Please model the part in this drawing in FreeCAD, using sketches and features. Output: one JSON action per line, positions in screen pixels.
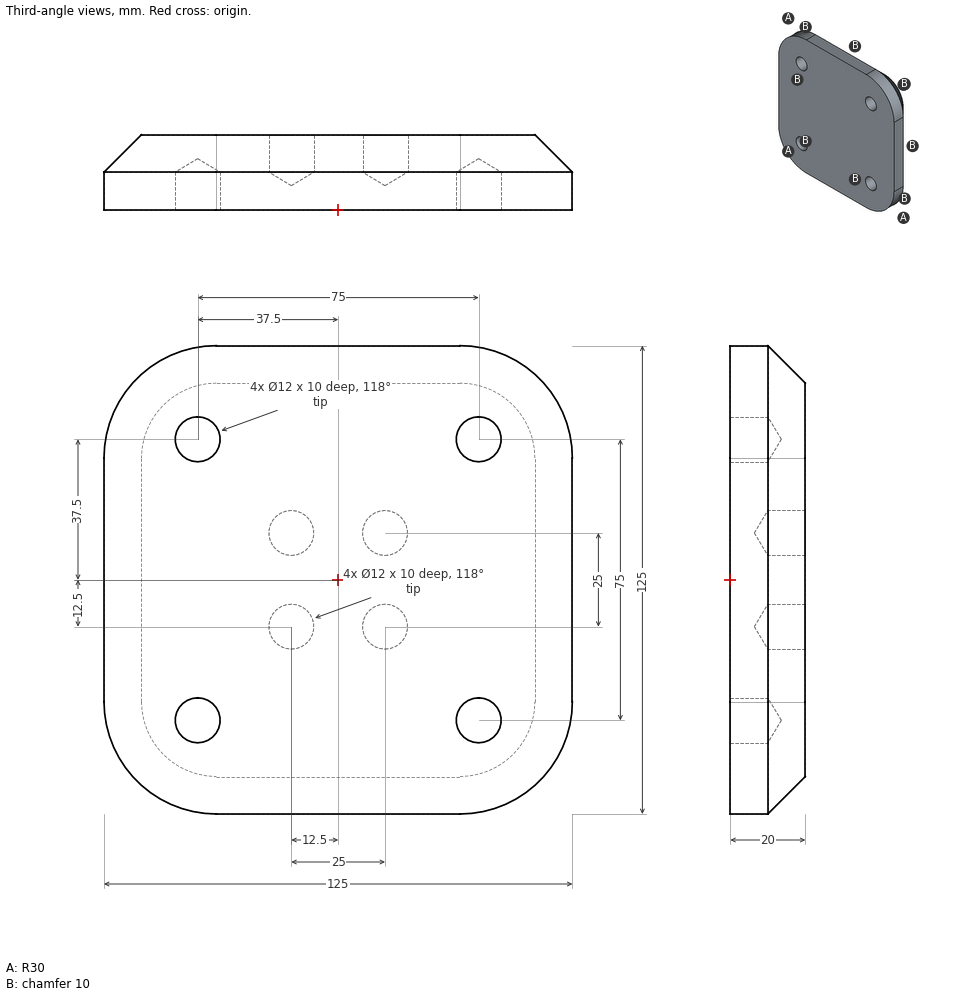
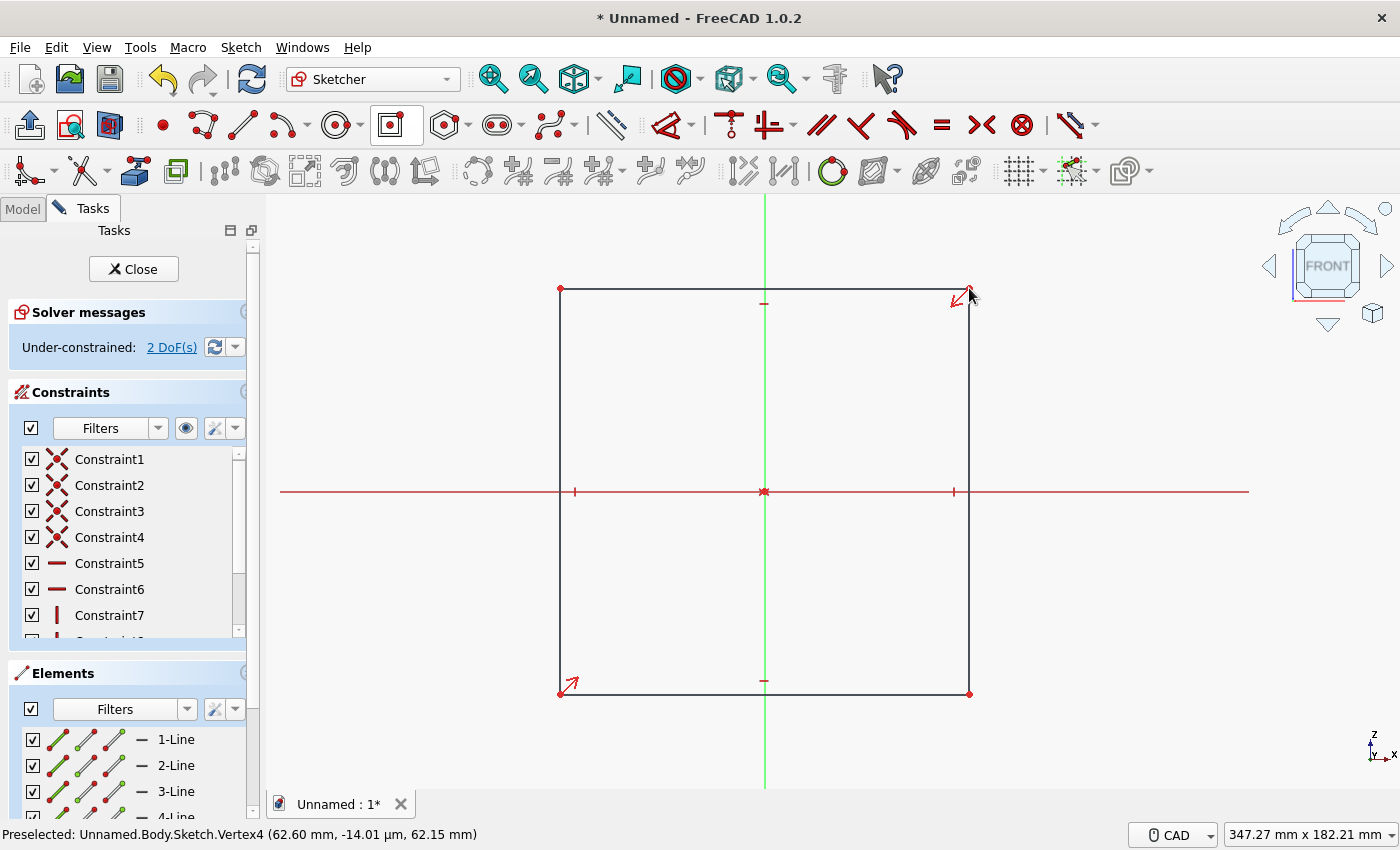
{"action": "key", "text": "d"}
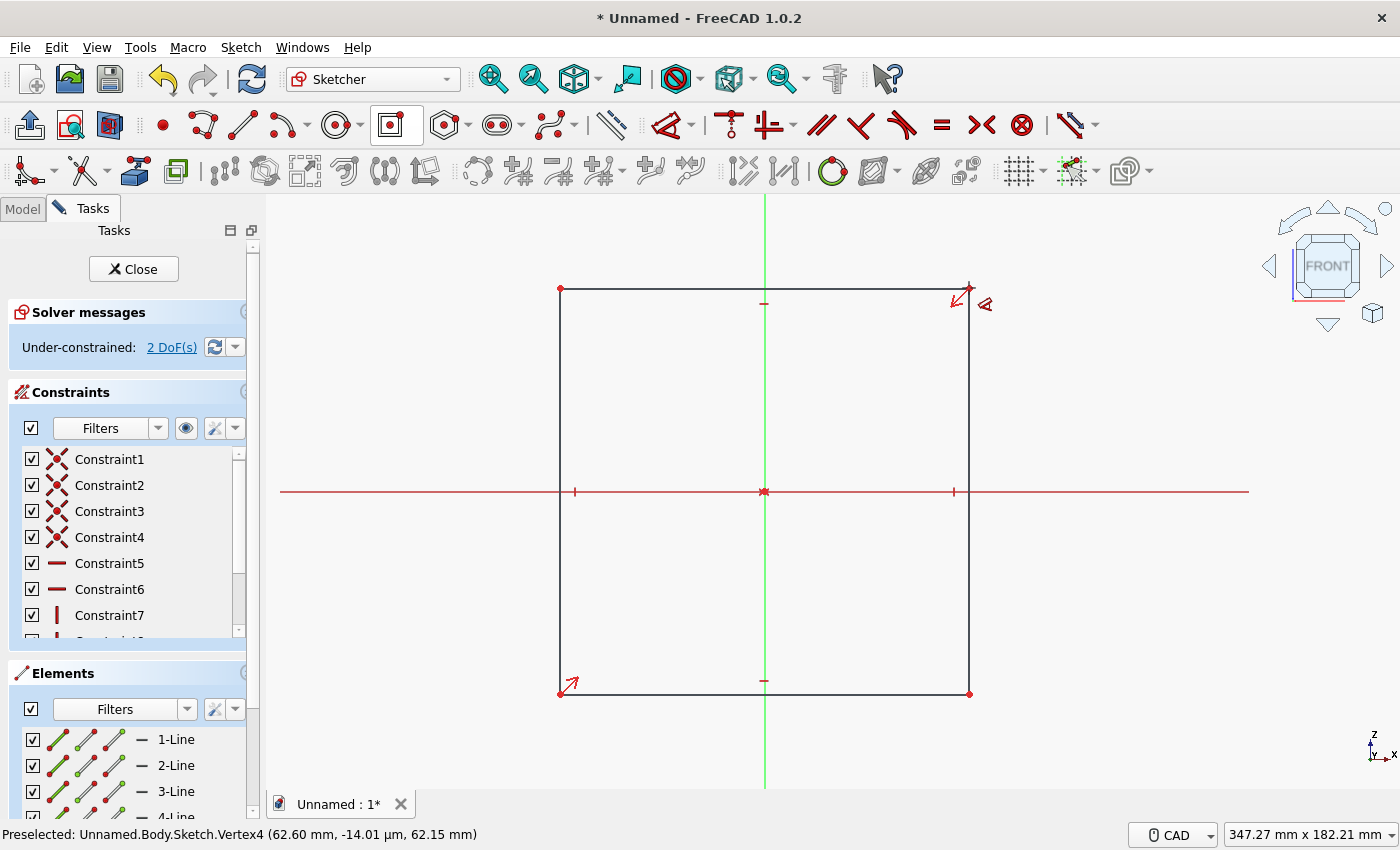
{"action": "left_click", "coordinate": [683, 695]}
{"action": "left_click", "coordinate": [671, 729]}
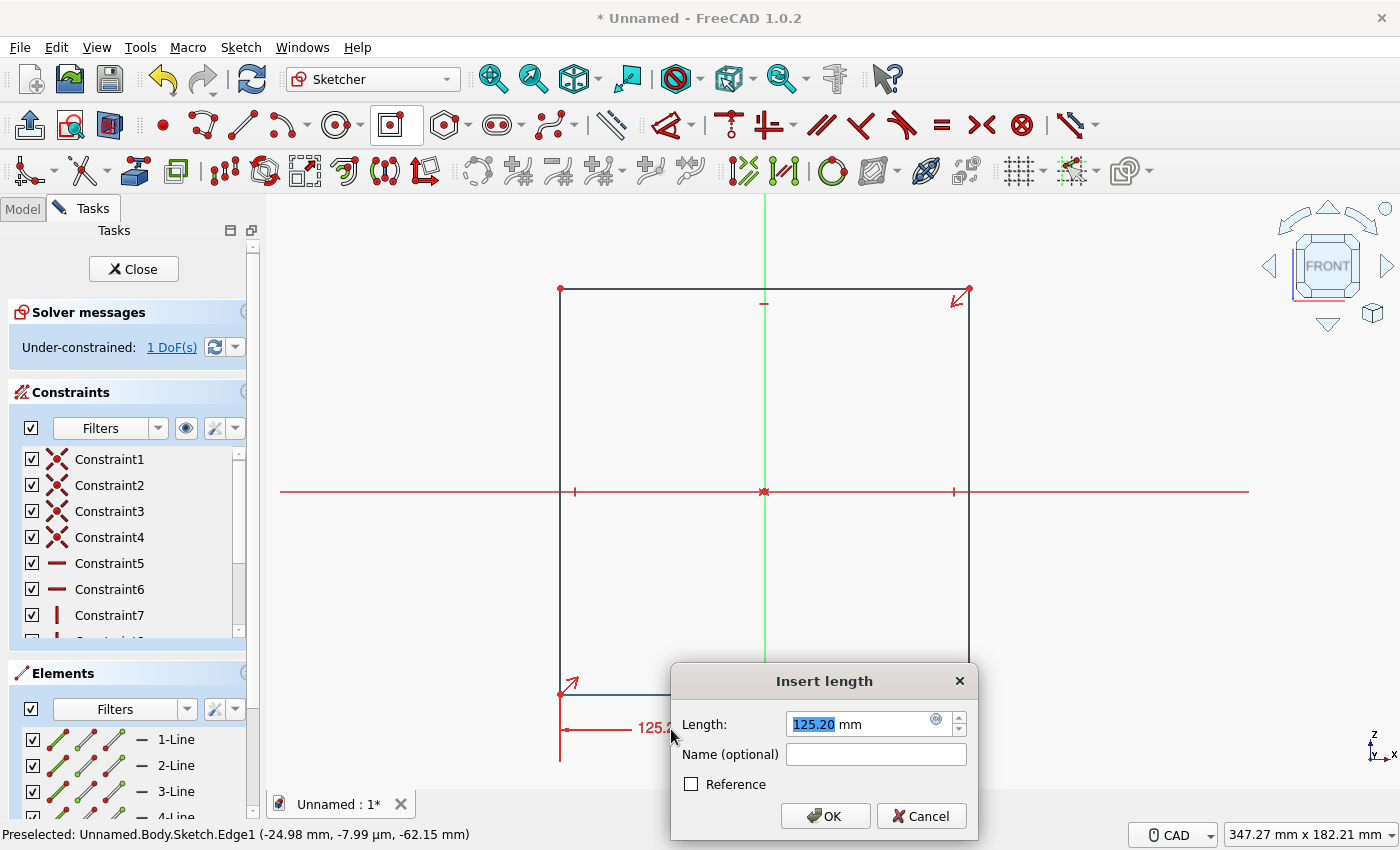
{"action": "type", "text": "125"}
{"action": "key", "text": "Return"}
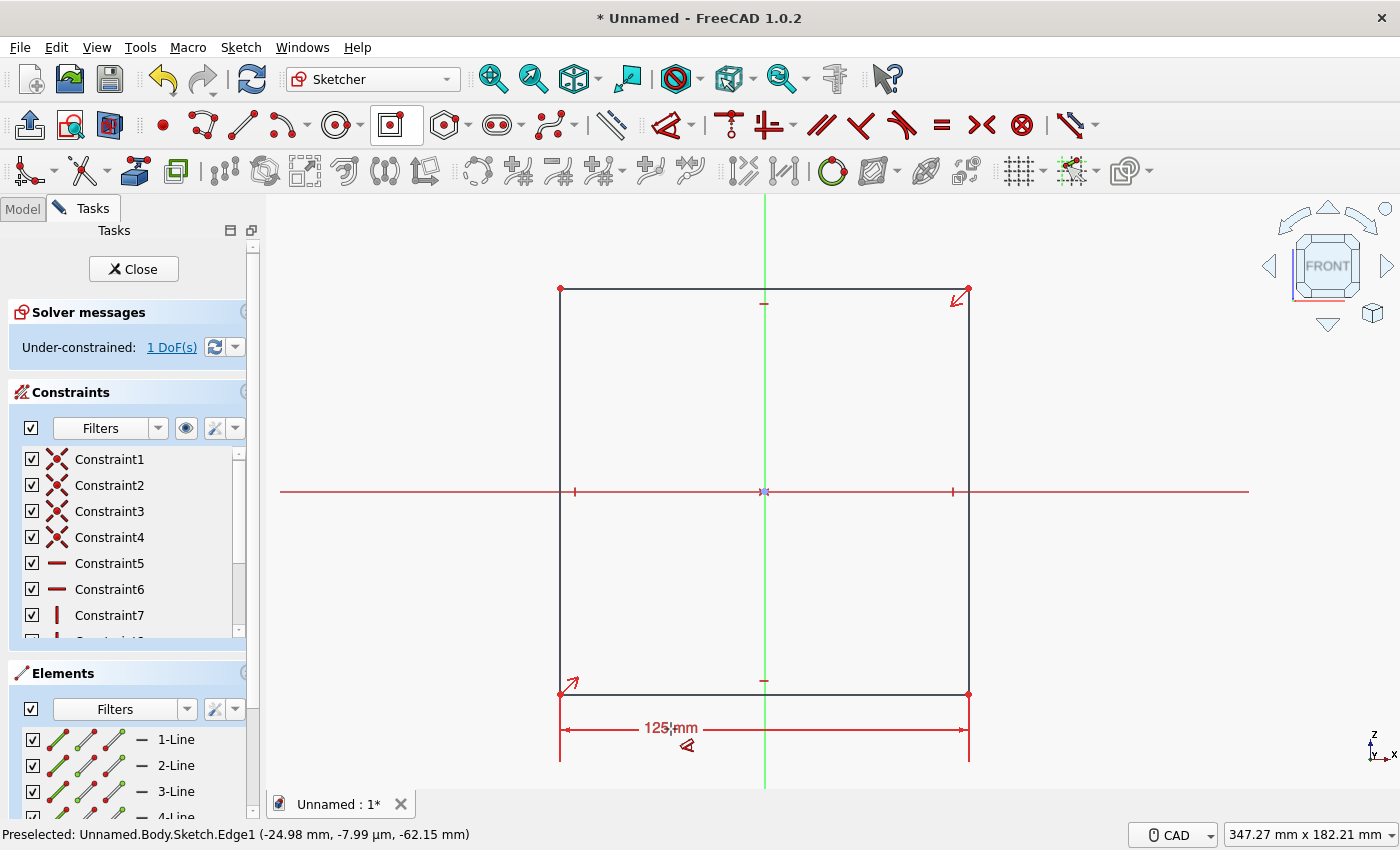
{"action": "left_click", "coordinate": [969, 573]}
{"action": "left_click", "coordinate": [1003, 399]}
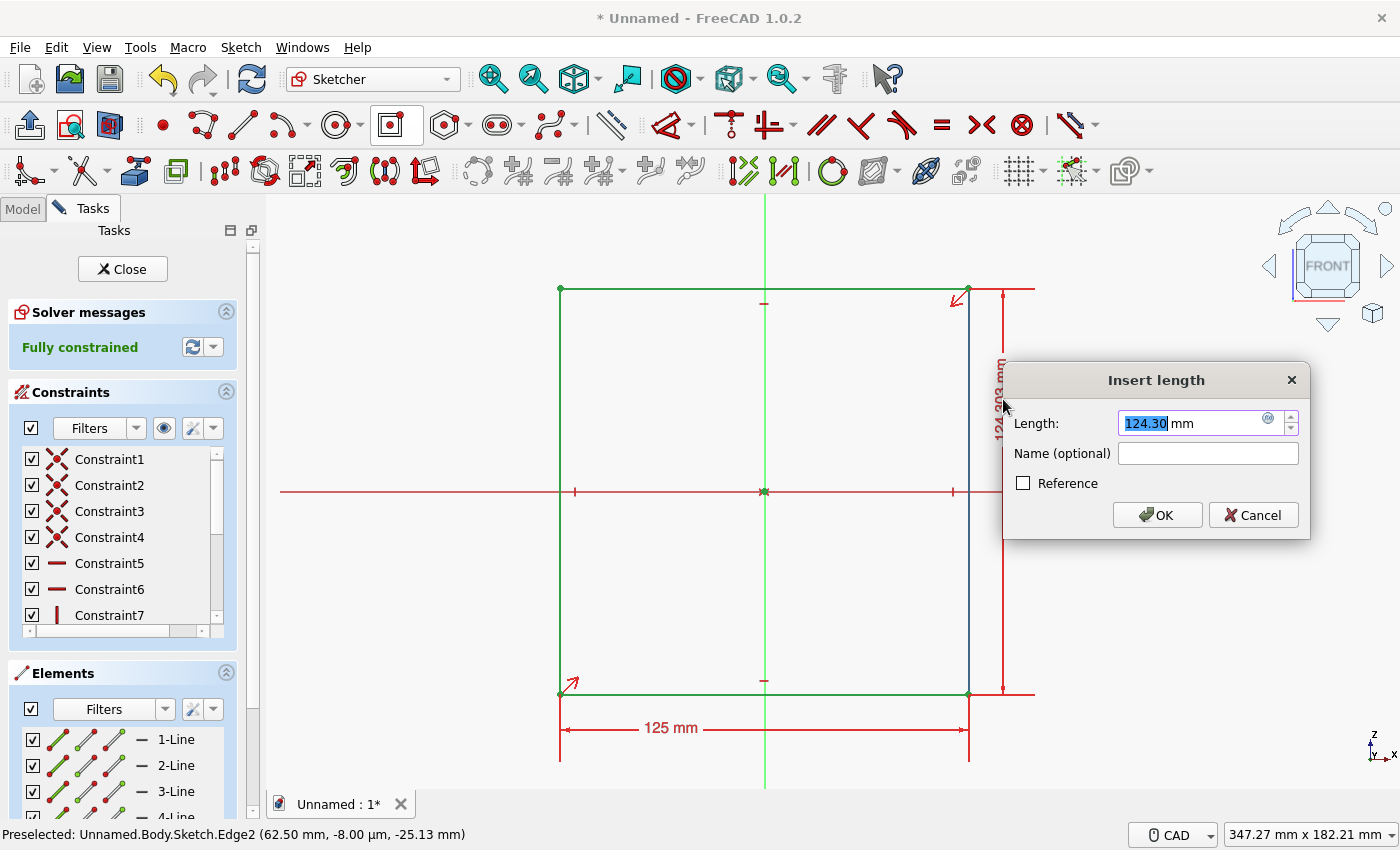
{"action": "type", "text": "125"}
{"action": "key", "text": "Return"}
{"action": "key", "text": "Escape"}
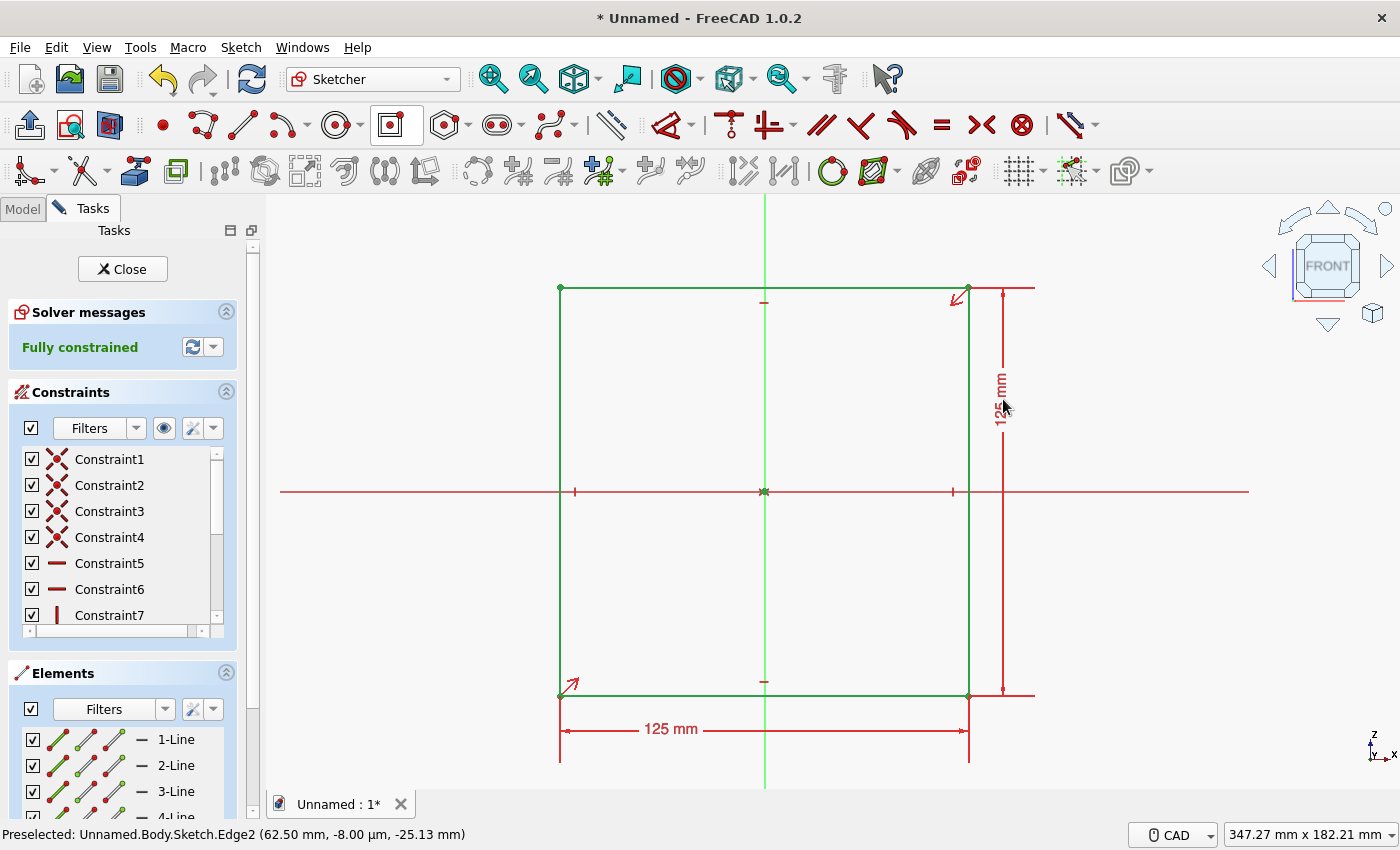
{"action": "left_click", "coordinate": [123, 269]}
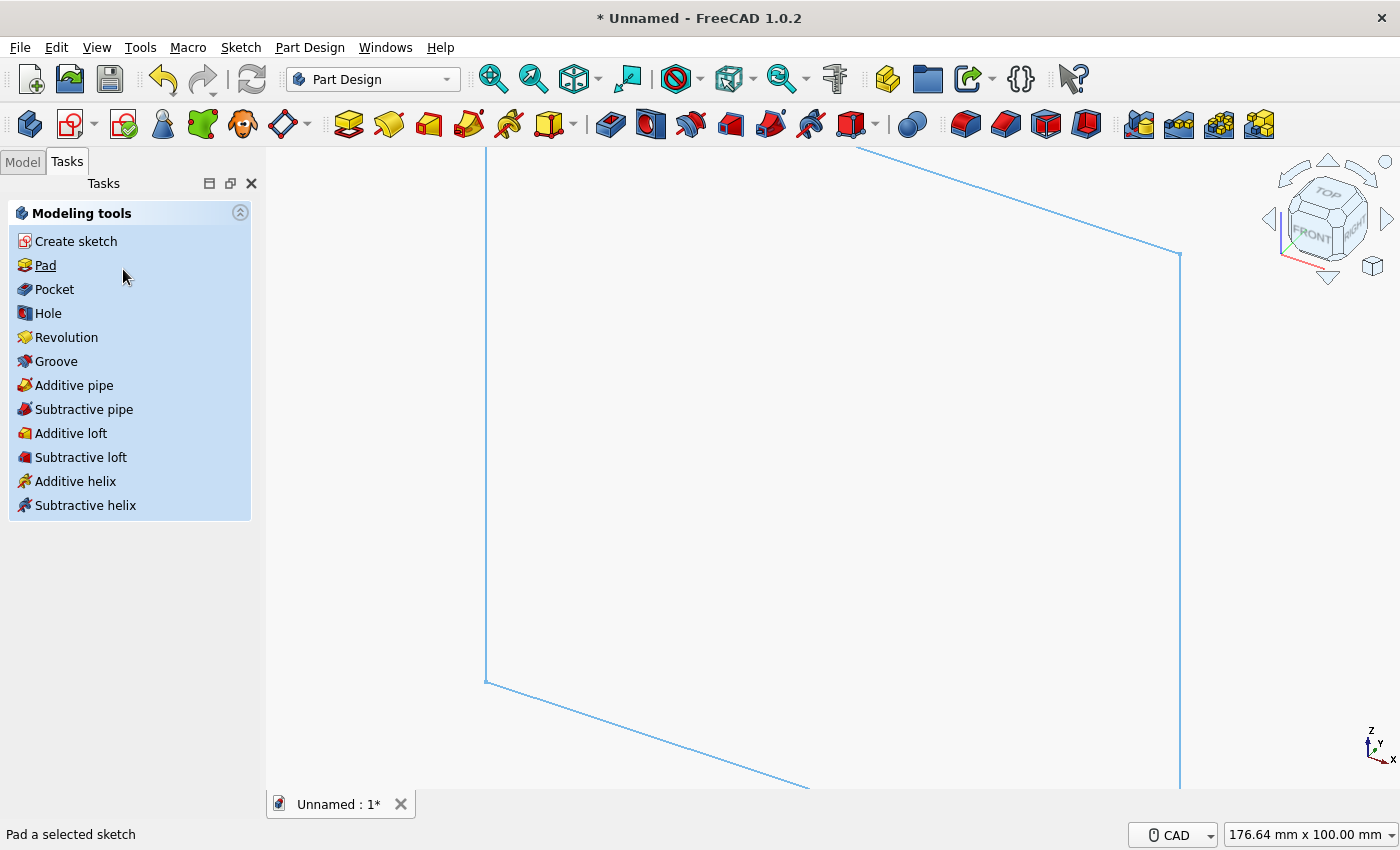
{"action": "left_click", "coordinate": [350, 124]}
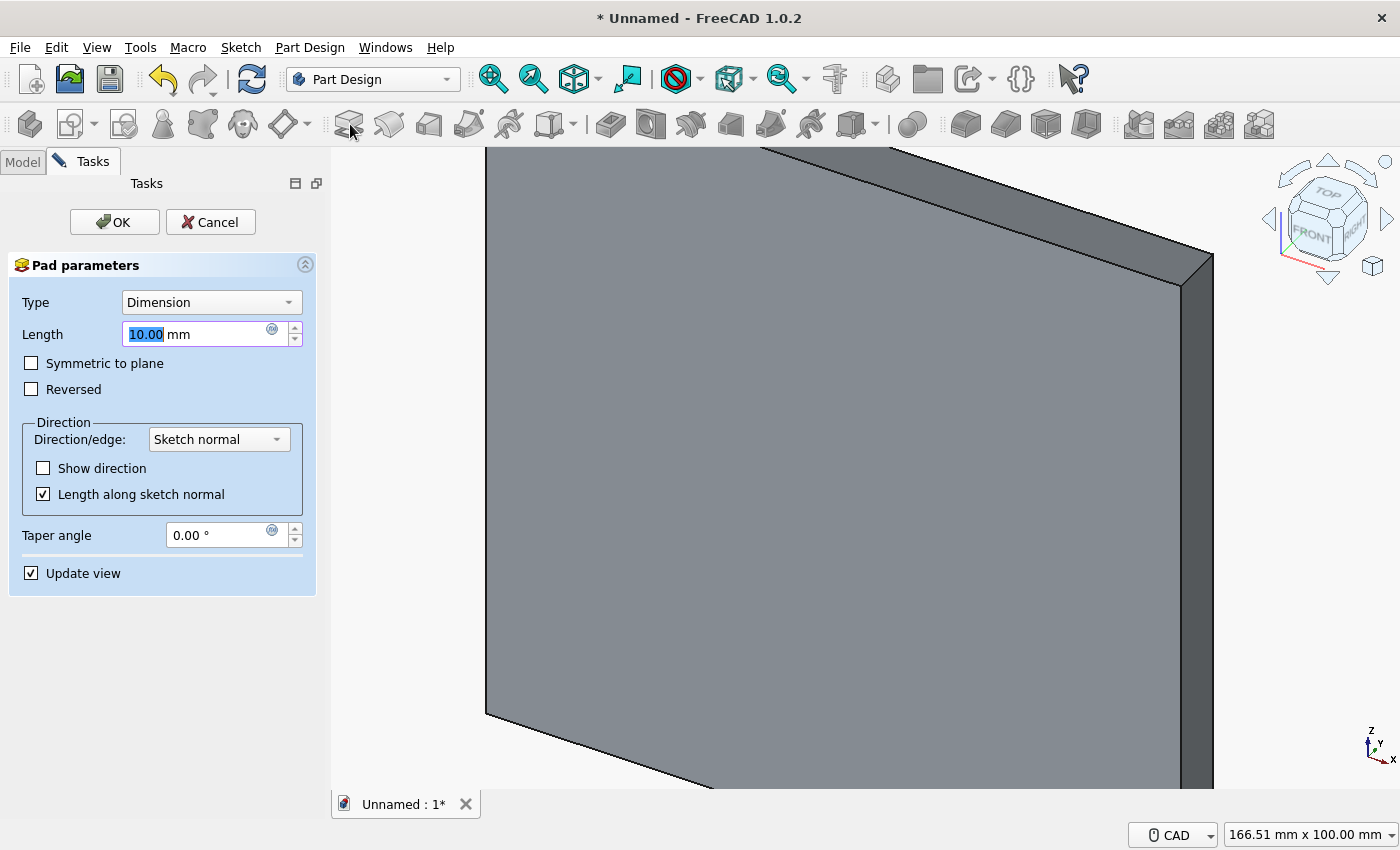
{"action": "type", "text": "20"}
{"action": "key", "text": "Tab"}